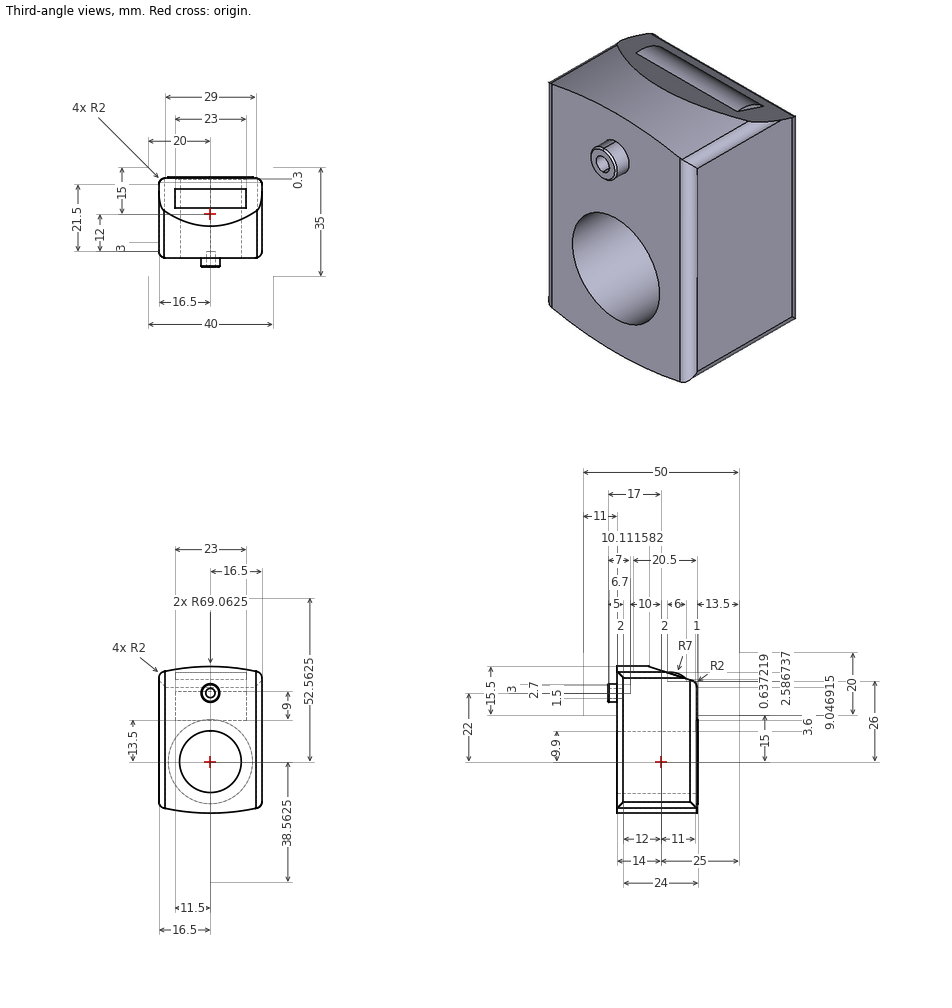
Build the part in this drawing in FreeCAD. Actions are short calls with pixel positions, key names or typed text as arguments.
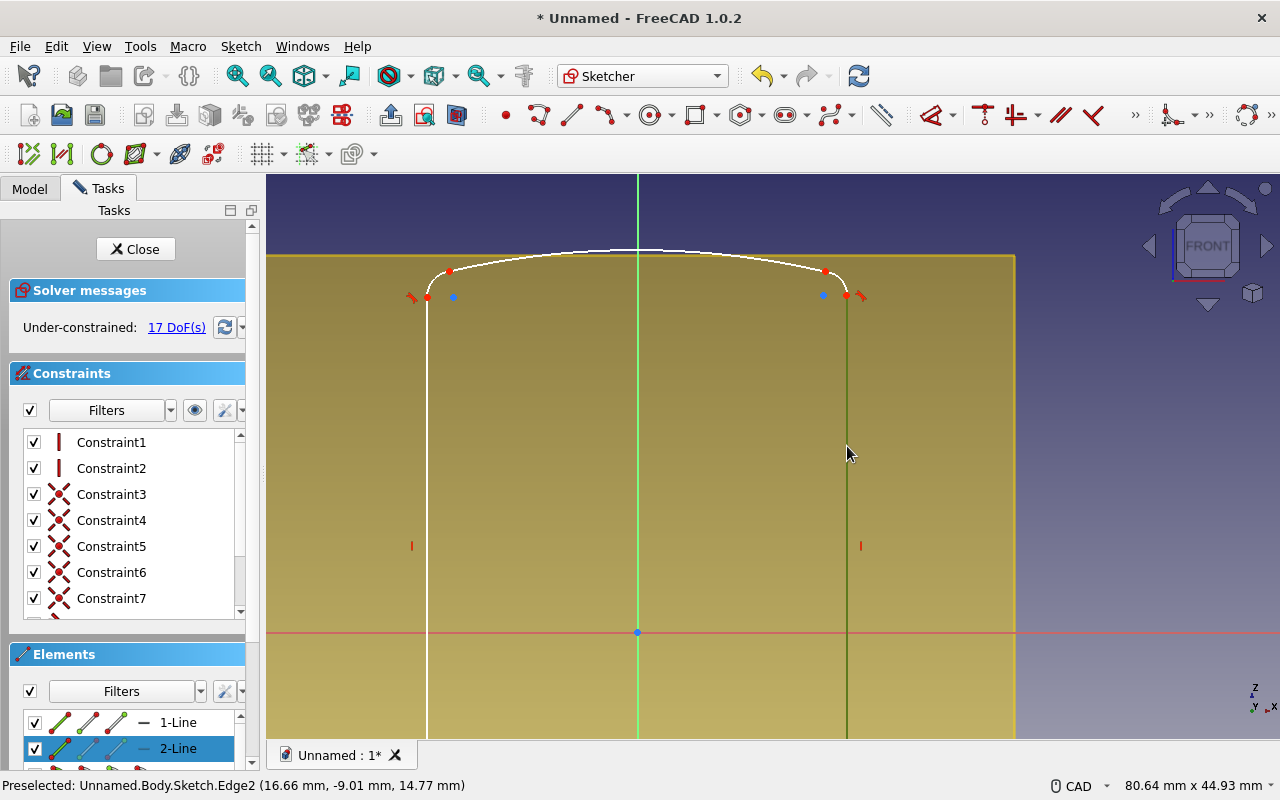
scroll(841, 277, down, 2)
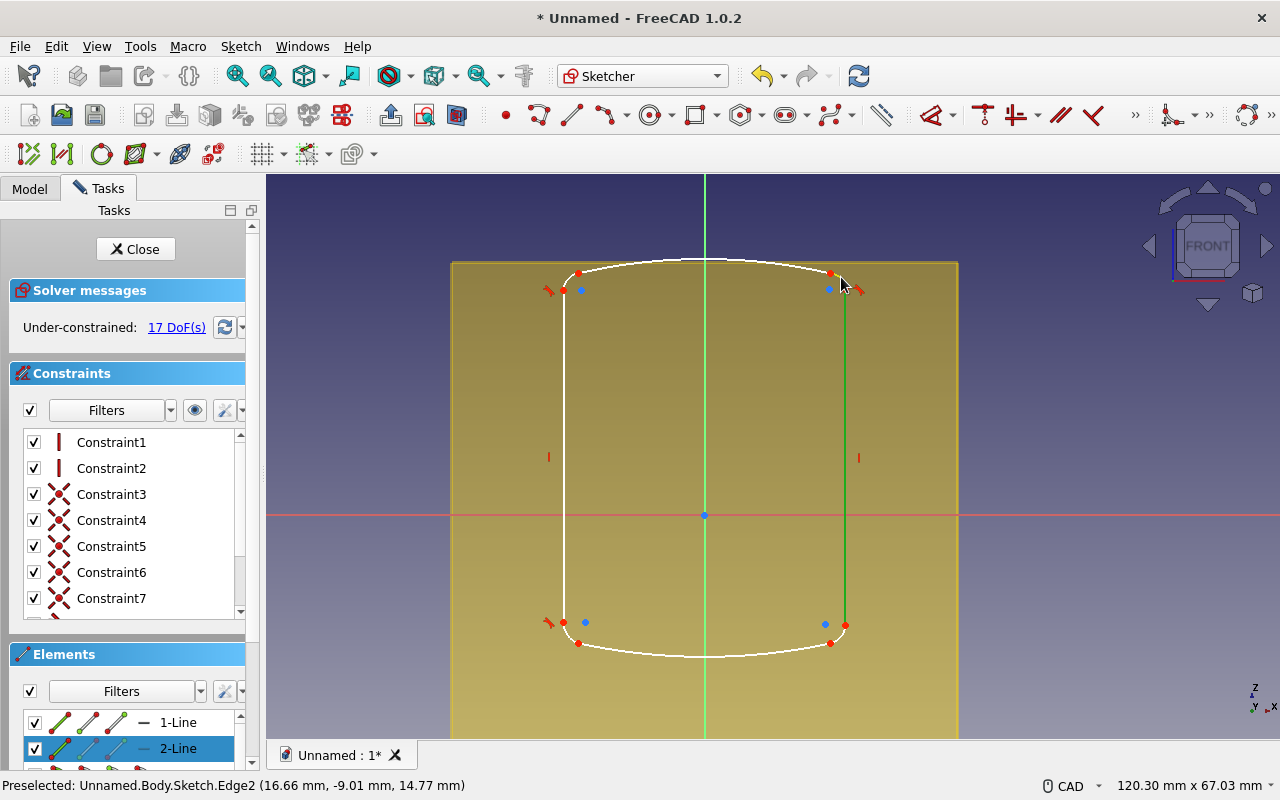
scroll(837, 640, up, 4)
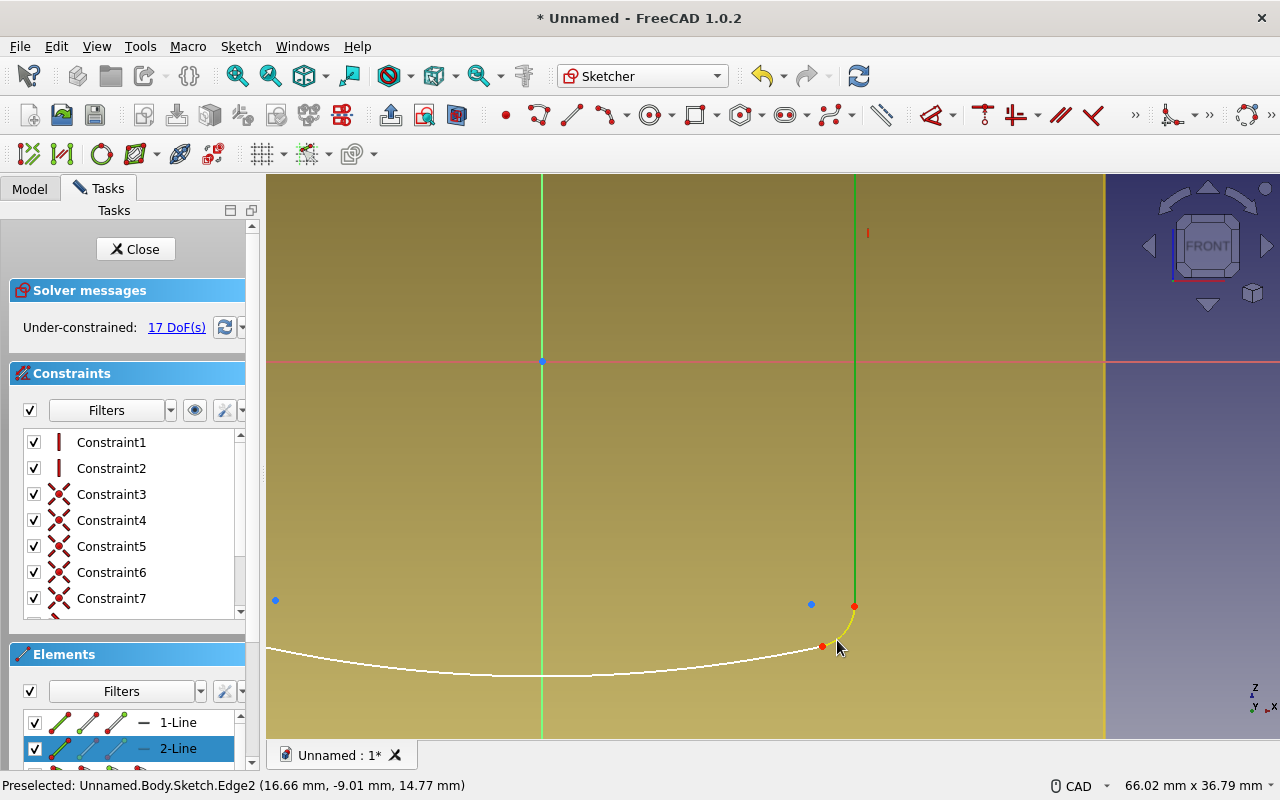
click(837, 639)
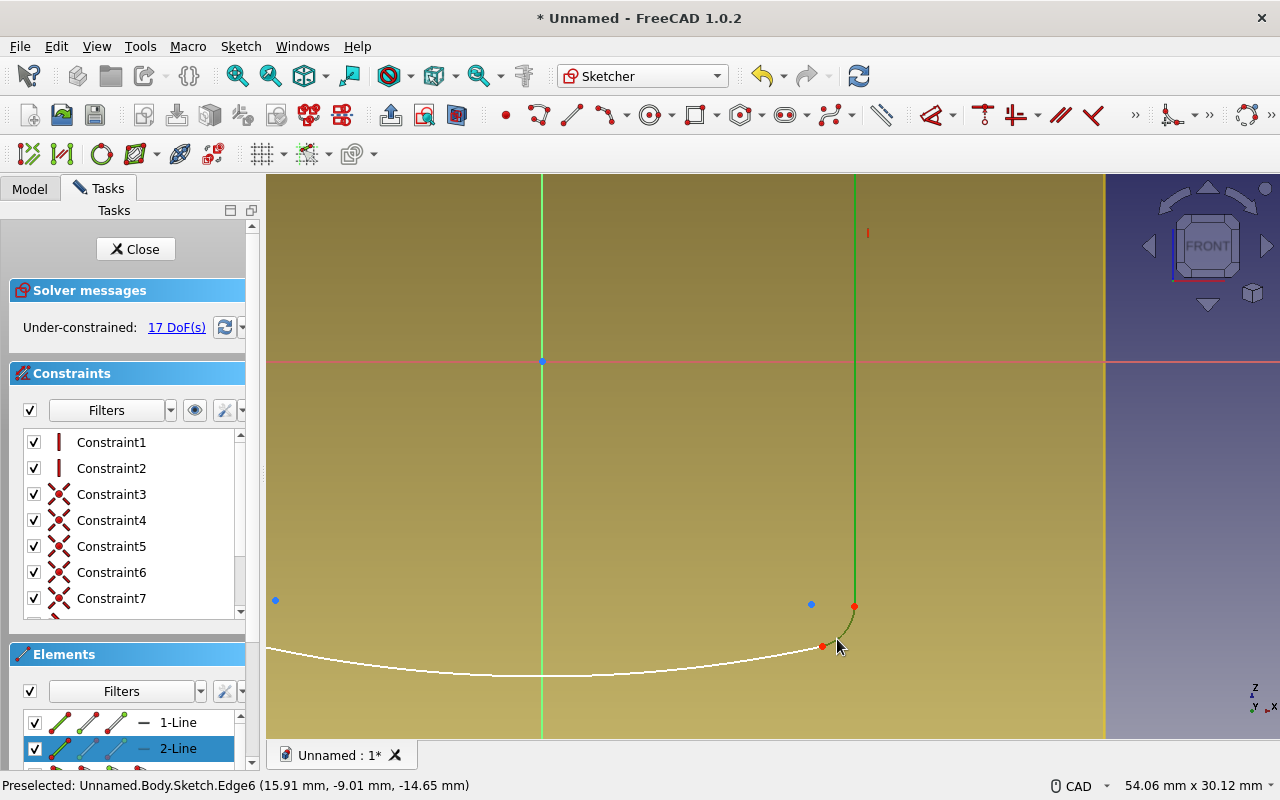
key(t)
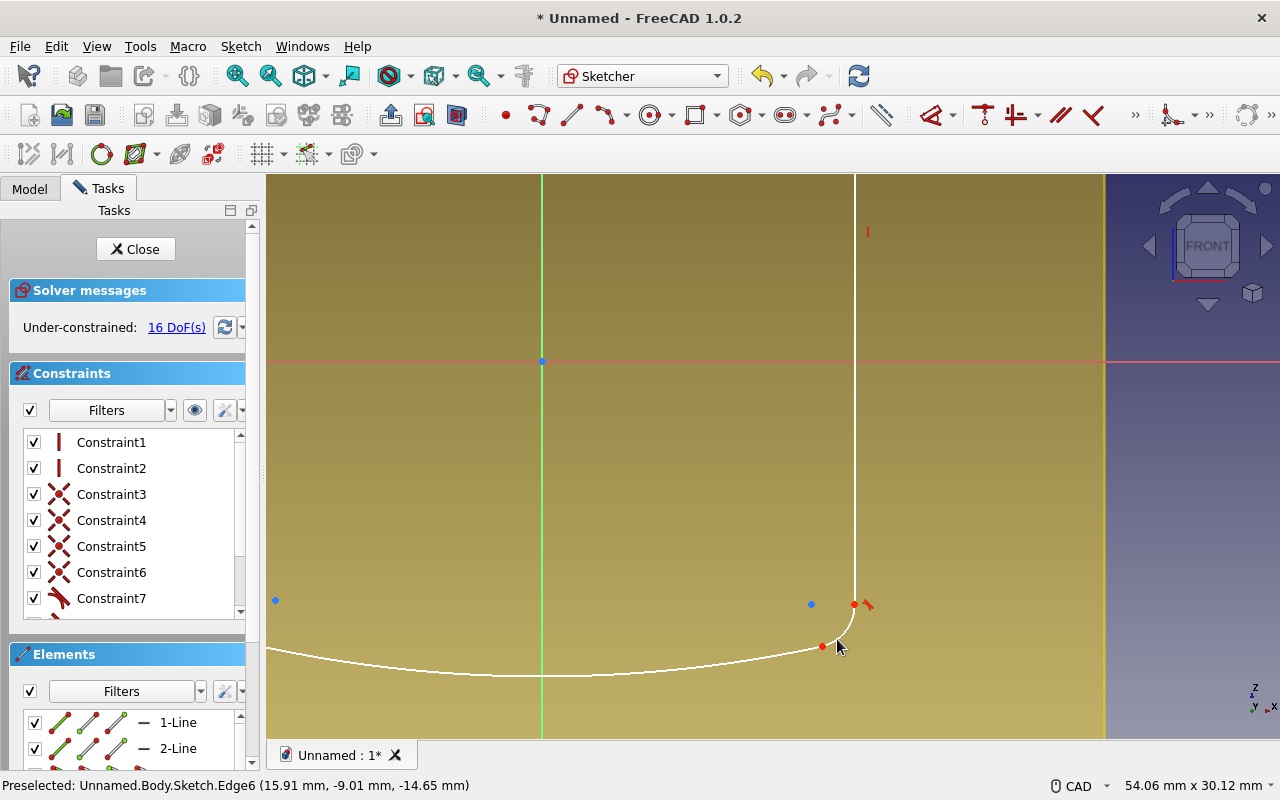
scroll(837, 641, down, 4)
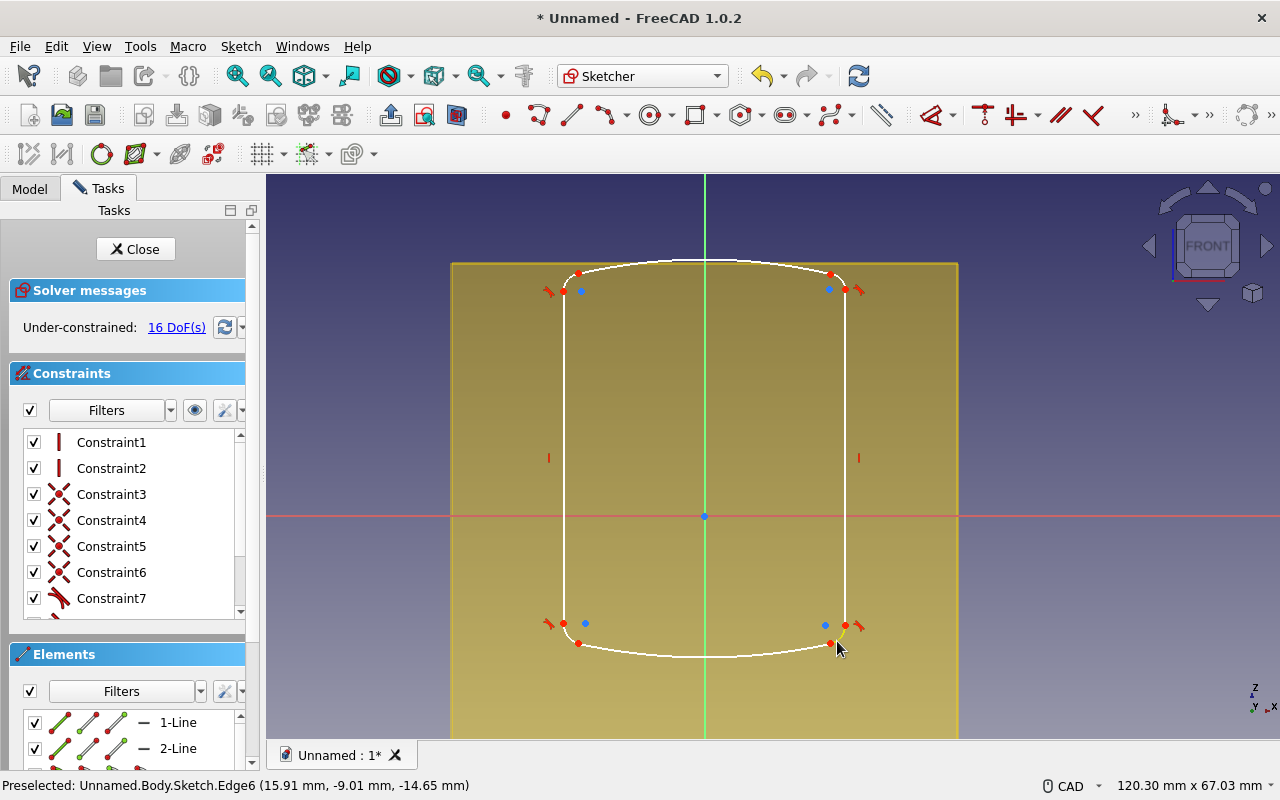
scroll(572, 277, up, 4)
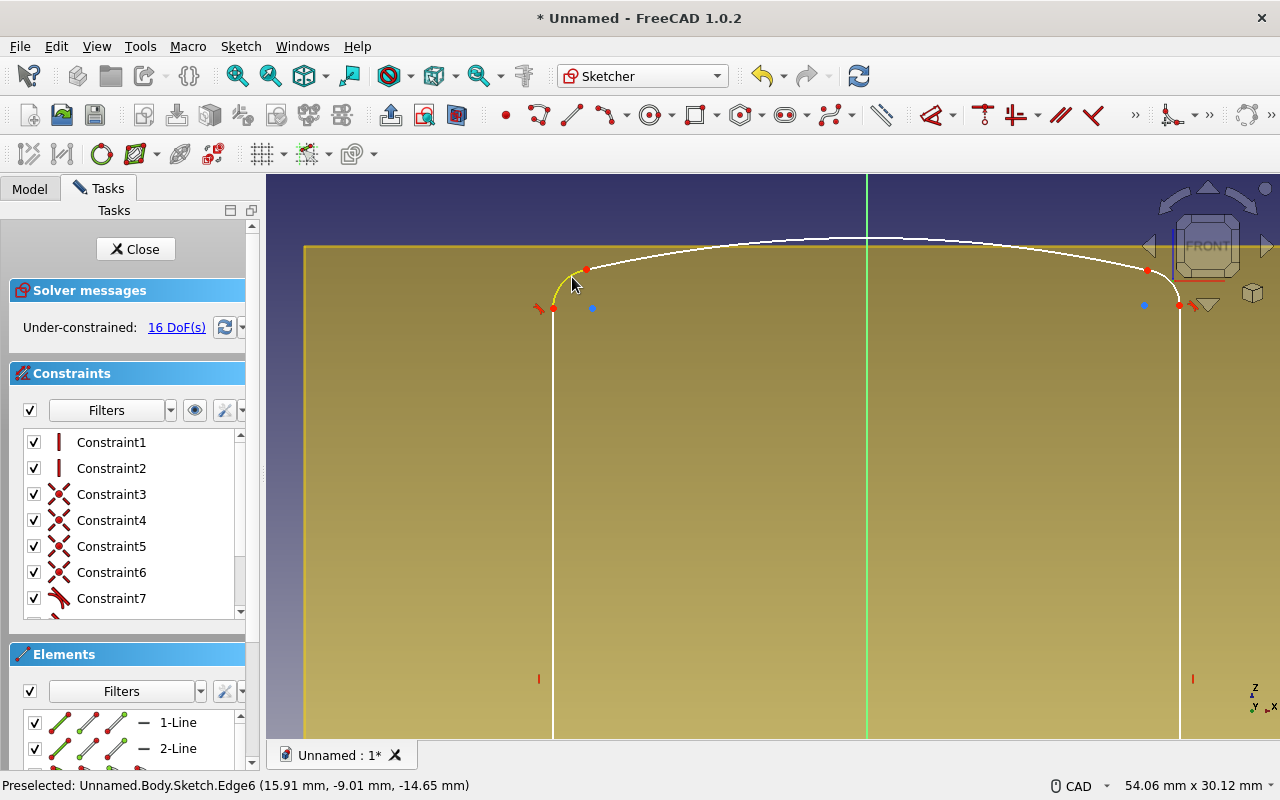
click(571, 276)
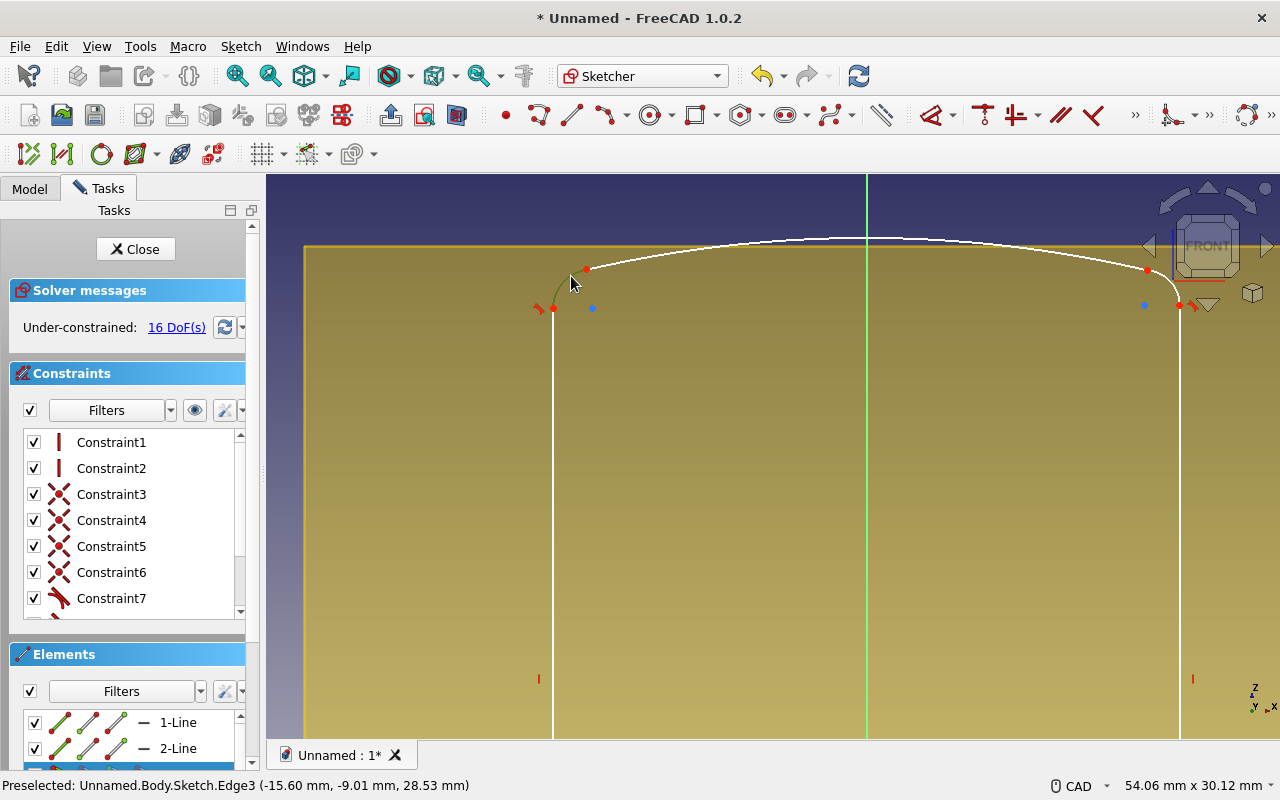
click(980, 243)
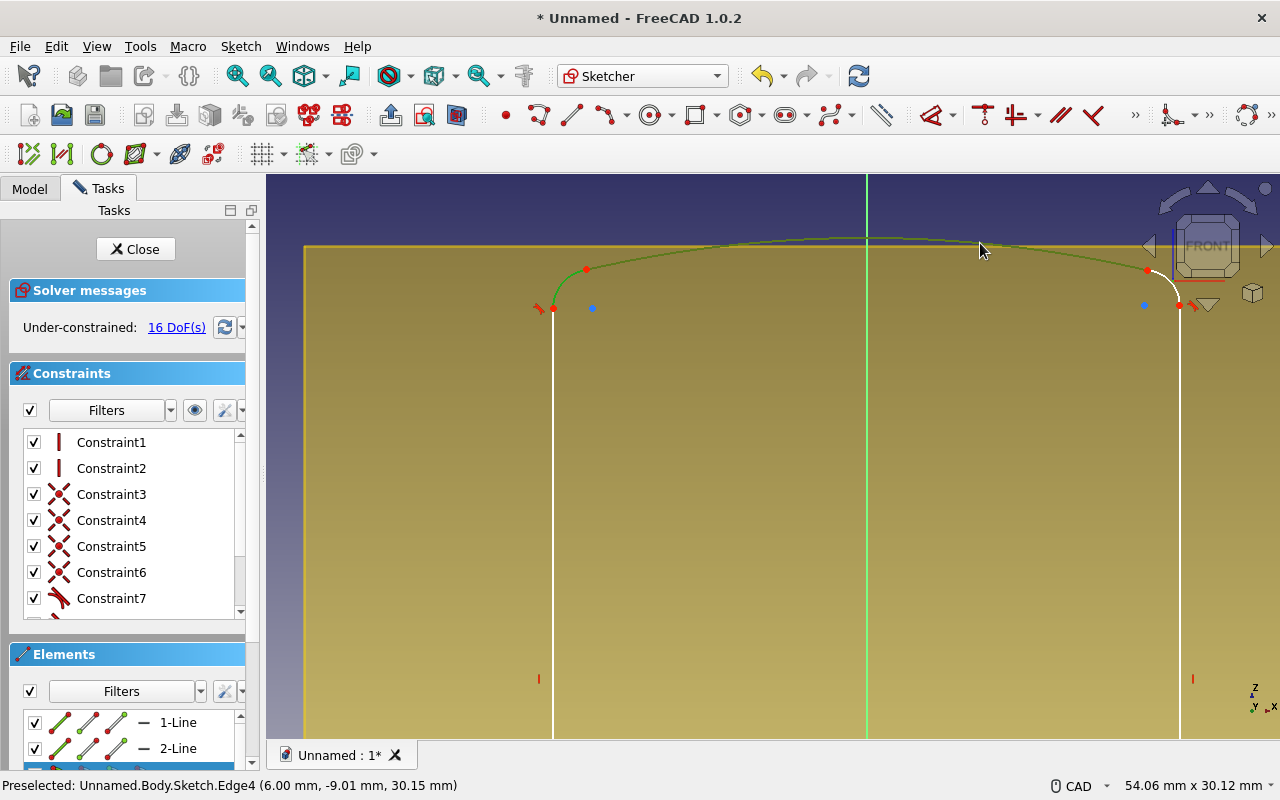
key(t)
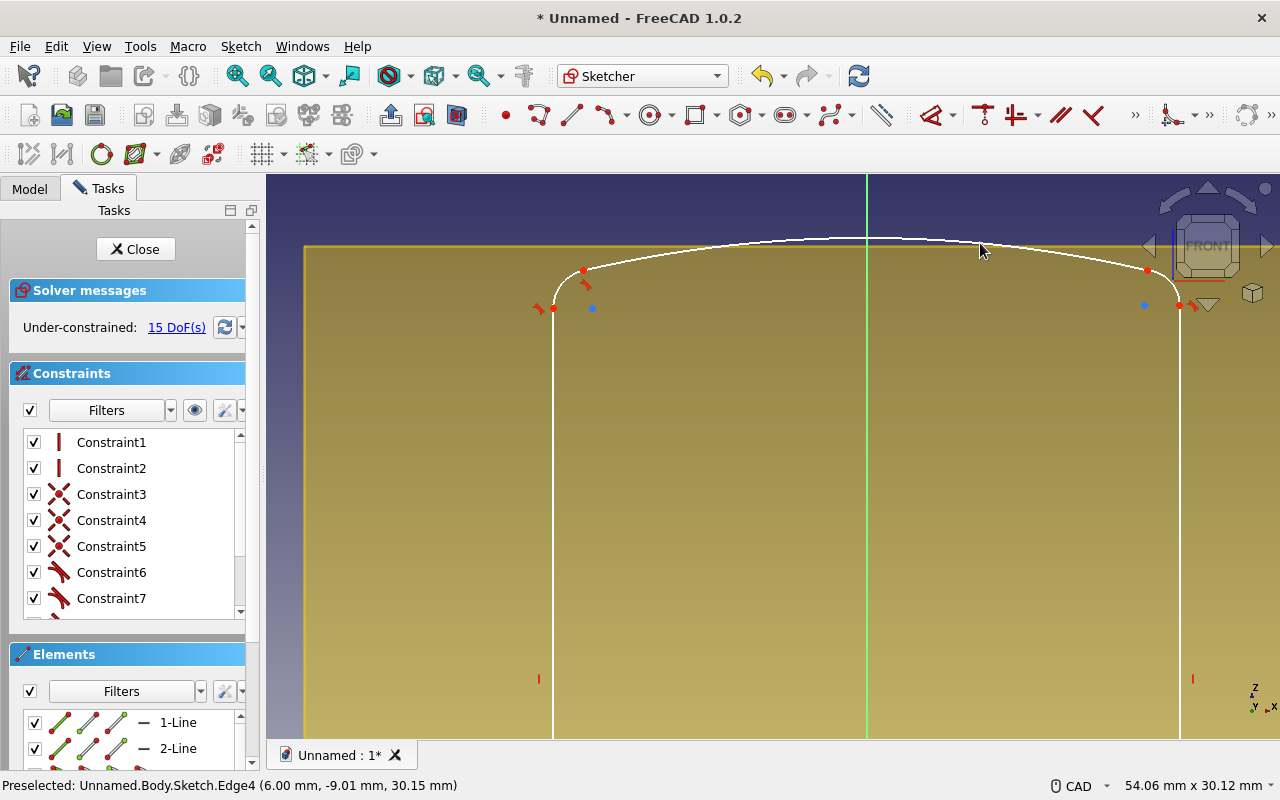
click(979, 243)